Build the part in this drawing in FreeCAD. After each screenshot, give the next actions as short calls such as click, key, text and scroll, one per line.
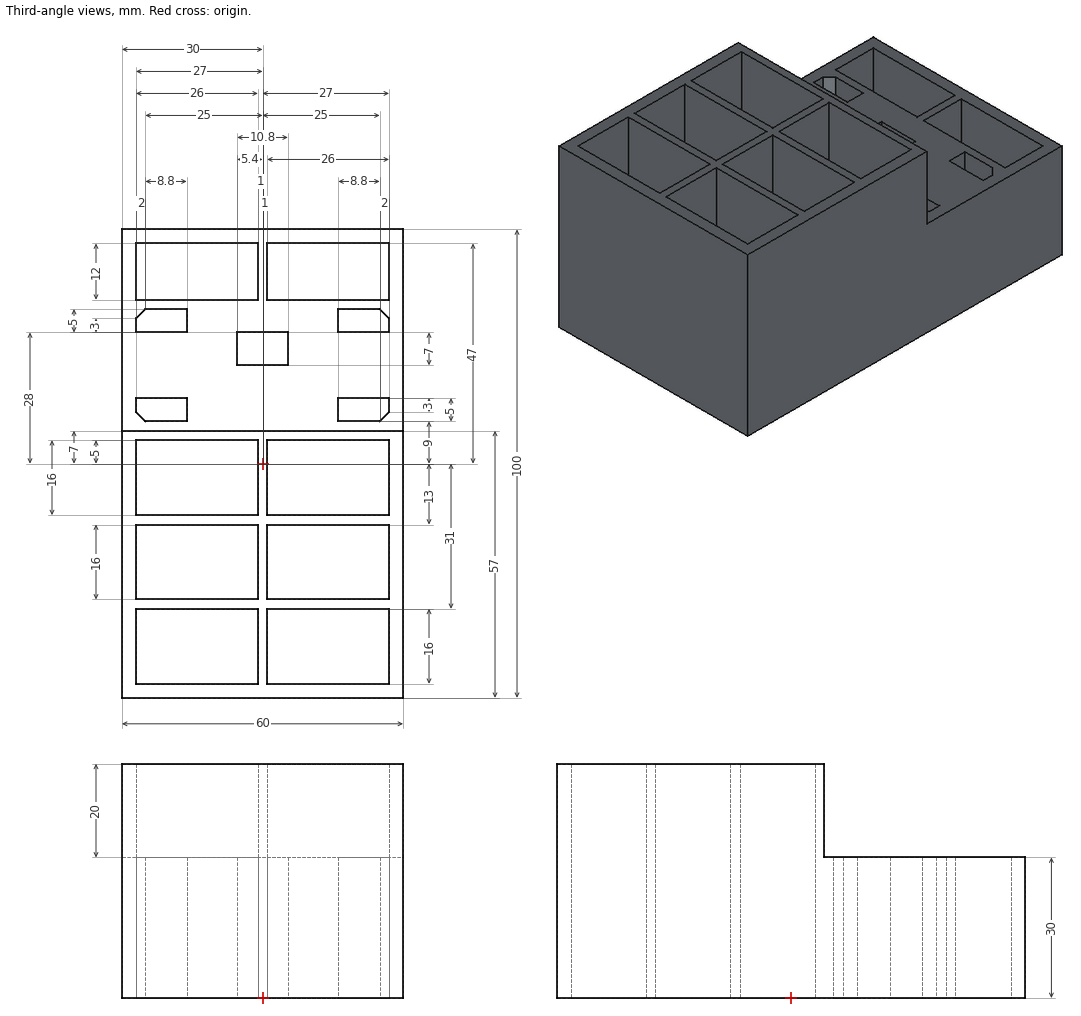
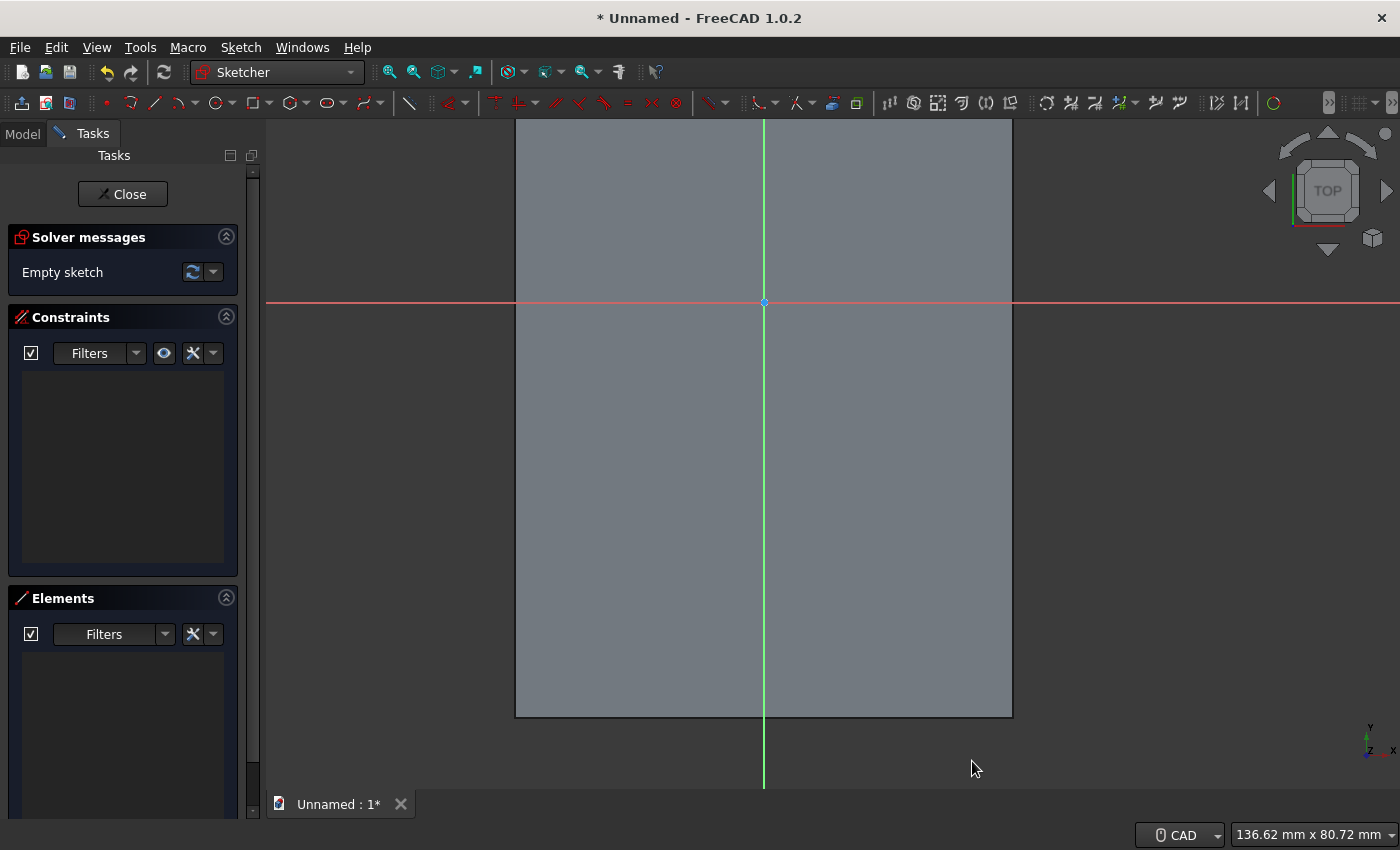
key(g)
key(r)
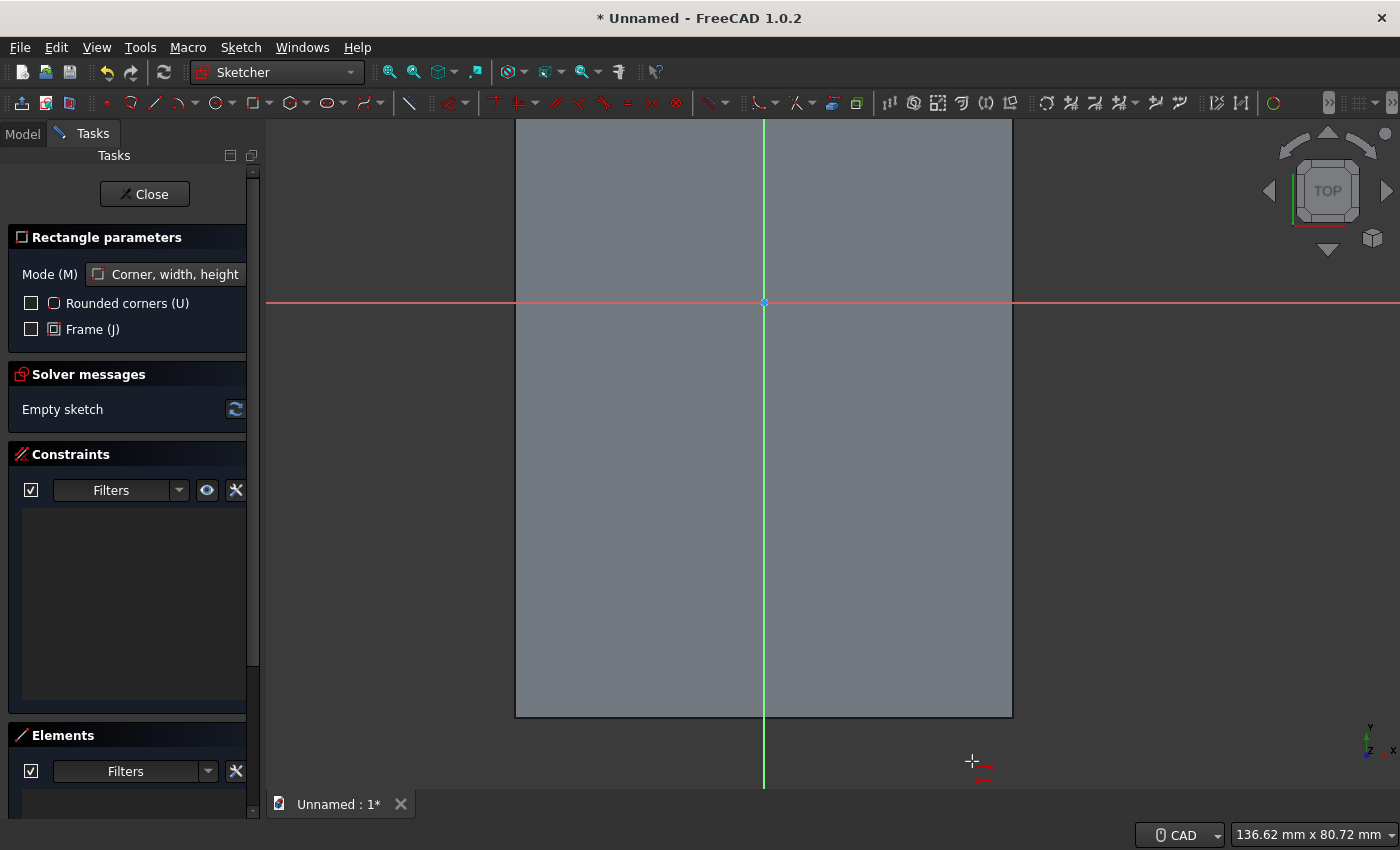
click(515, 244)
move(1013, 718)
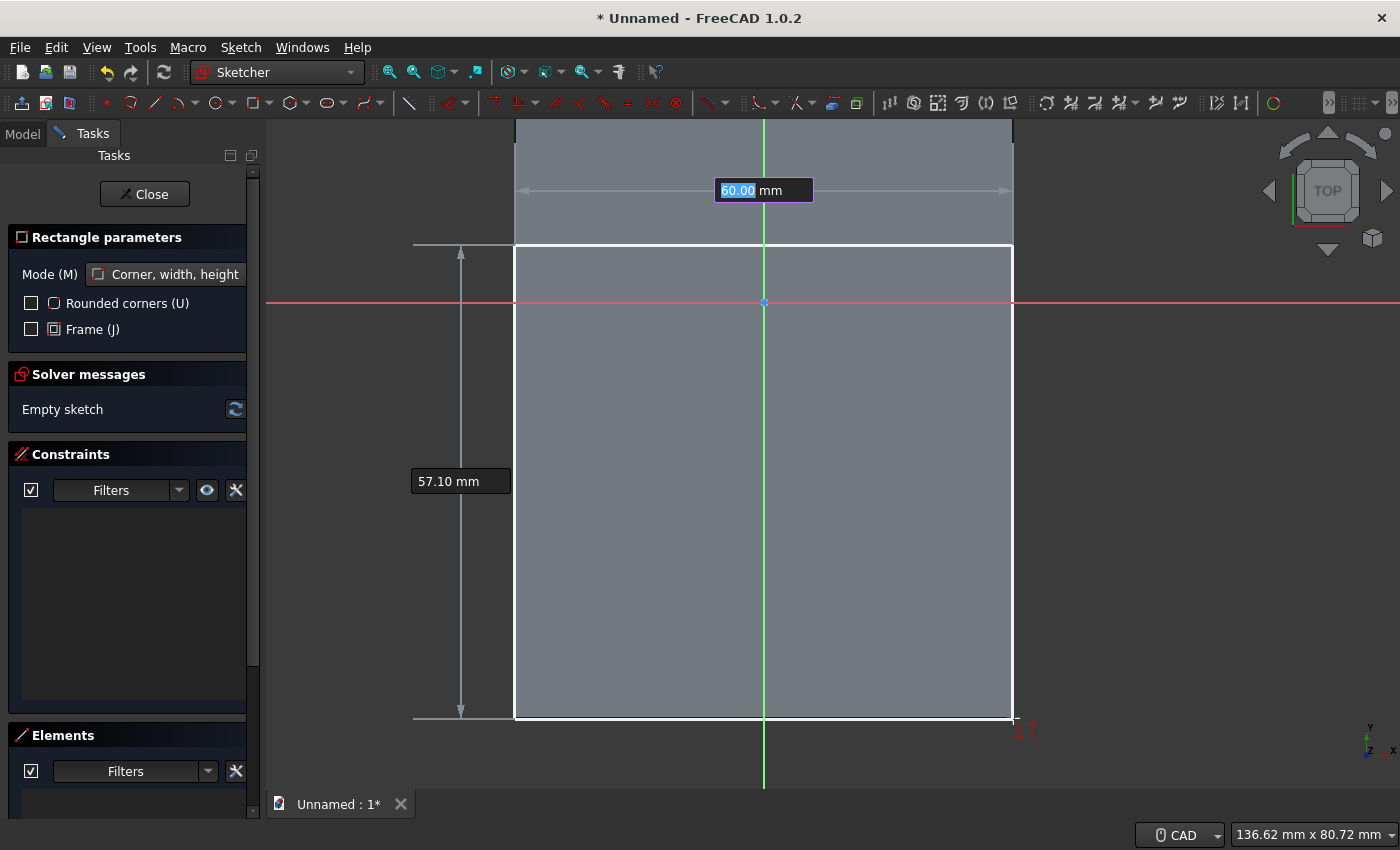
text(60)
key(Tab)
text(57)
key(Return)
key(Escape)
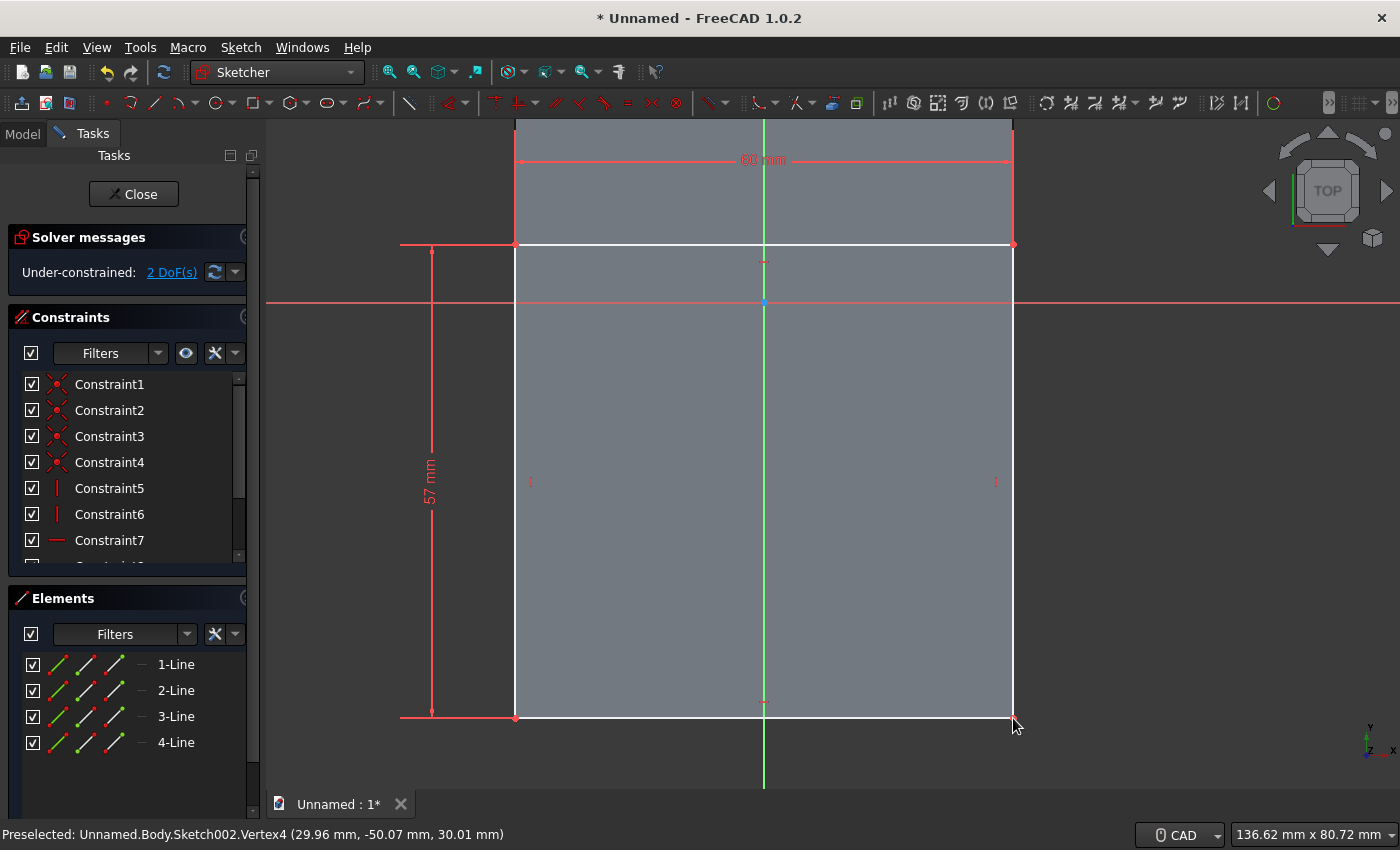
click(448, 104)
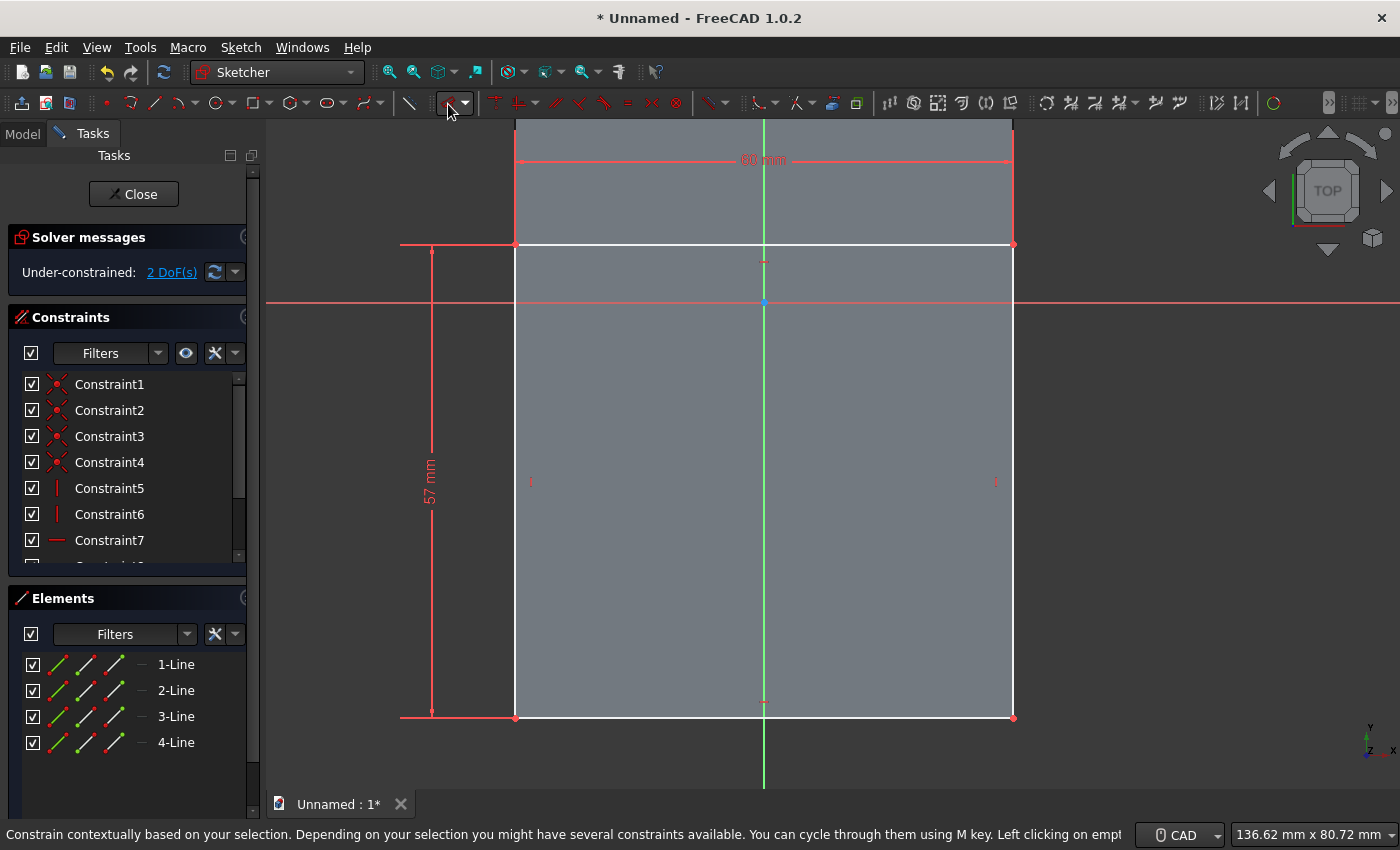
click(515, 245)
click(481, 274)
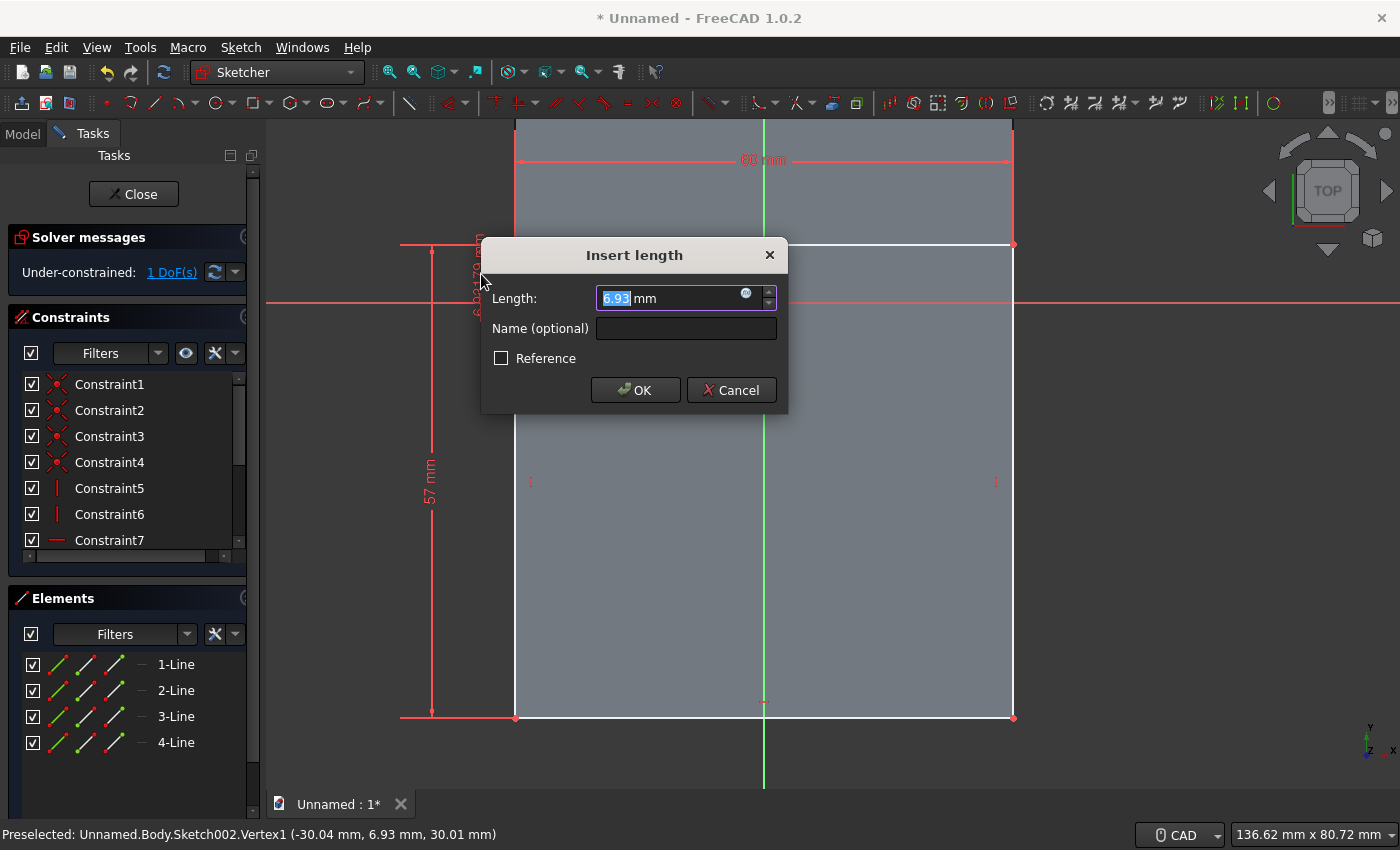
text(7)
key(Return)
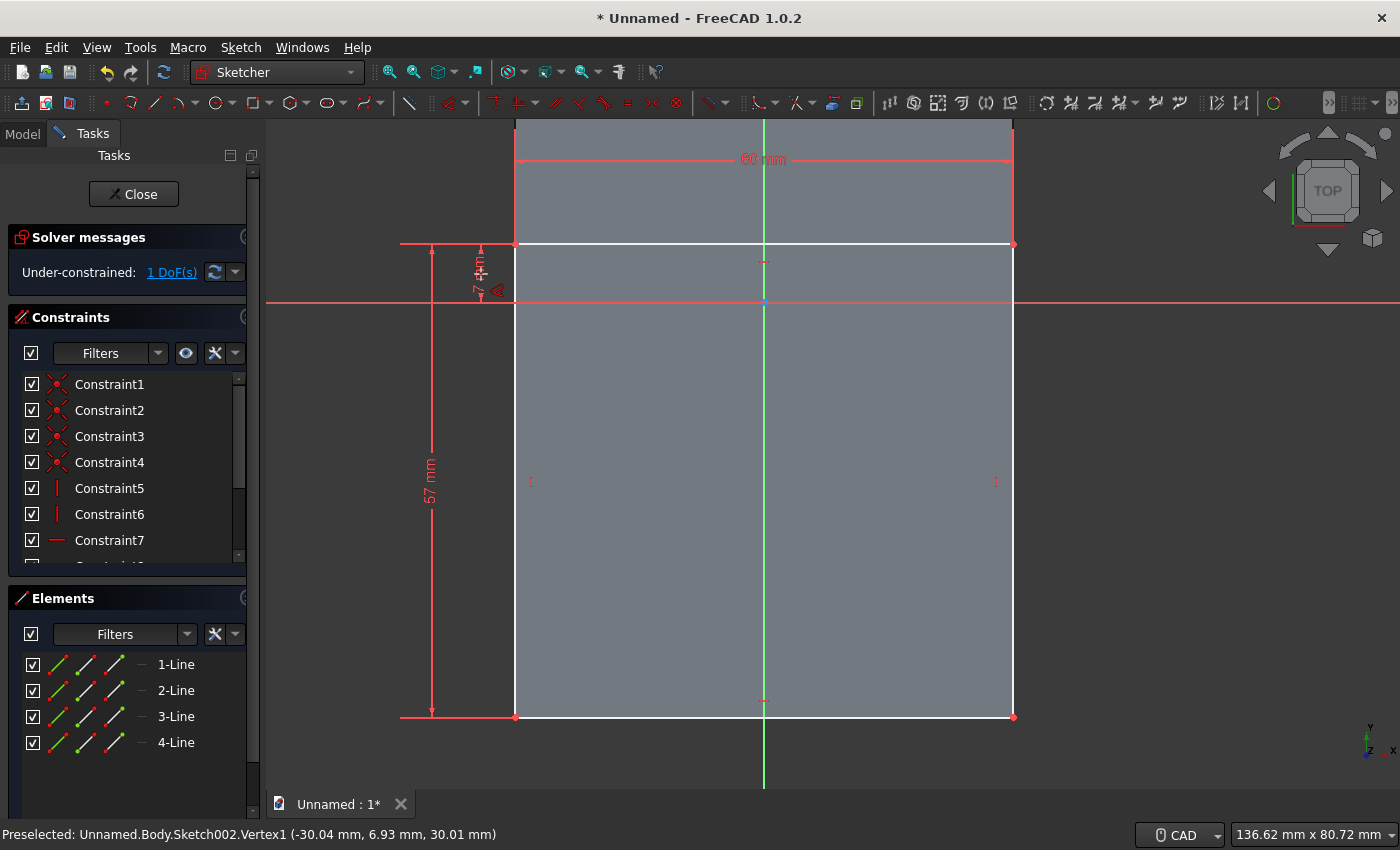
click(515, 244)
click(640, 210)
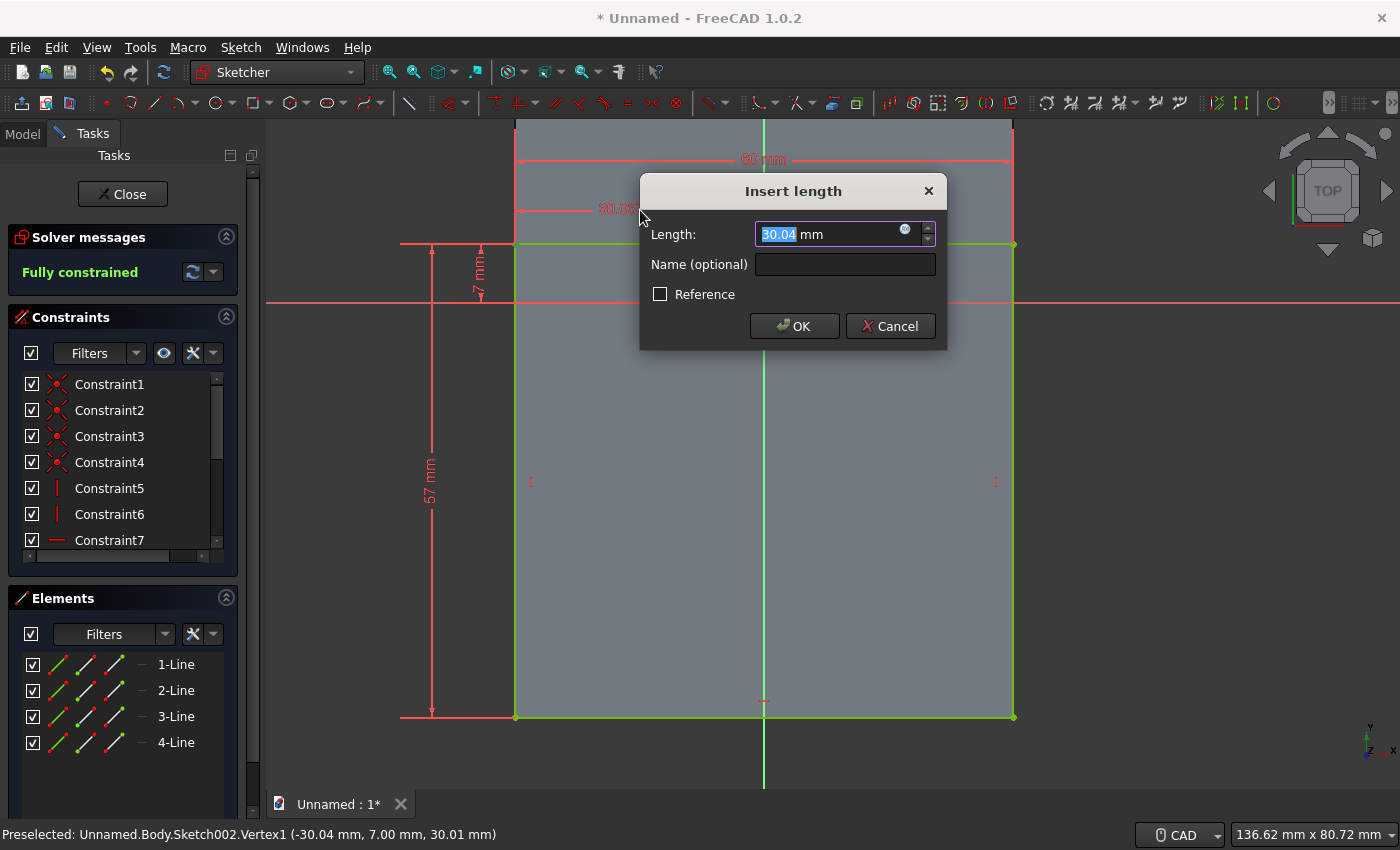
text(30)
key(Return)
key(Escape)